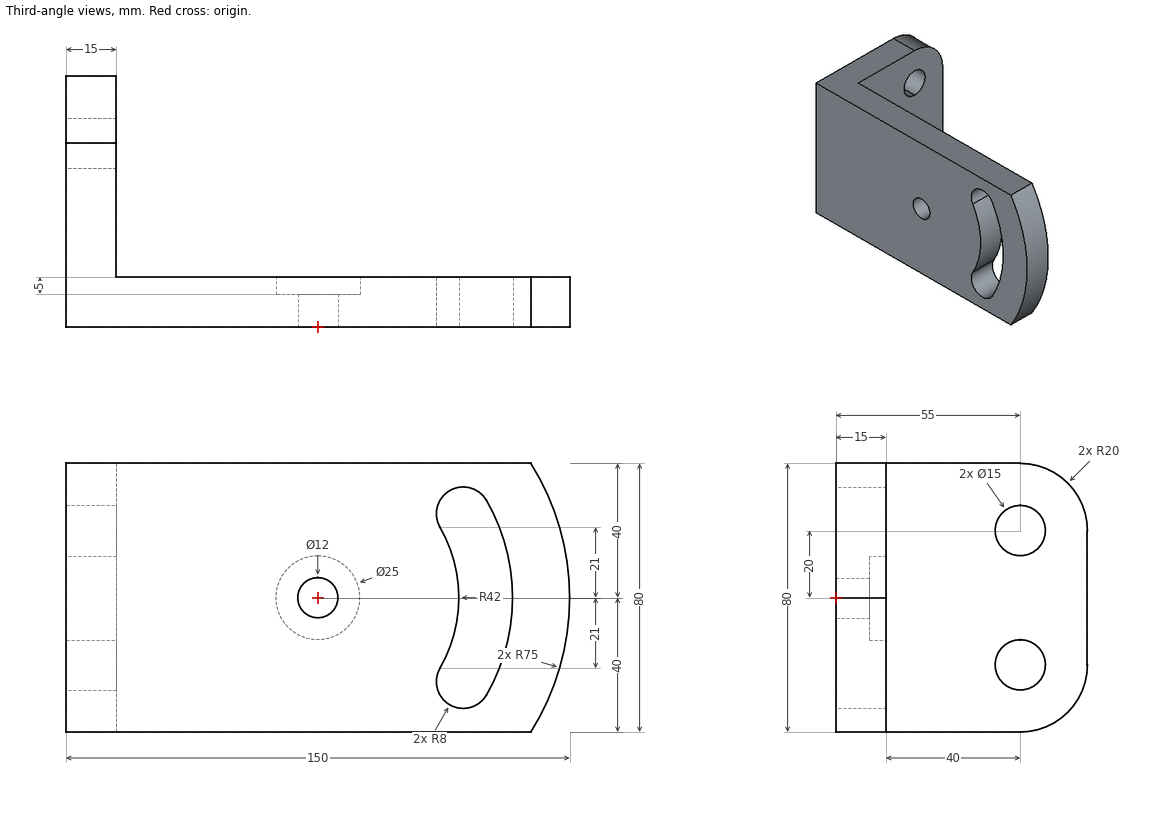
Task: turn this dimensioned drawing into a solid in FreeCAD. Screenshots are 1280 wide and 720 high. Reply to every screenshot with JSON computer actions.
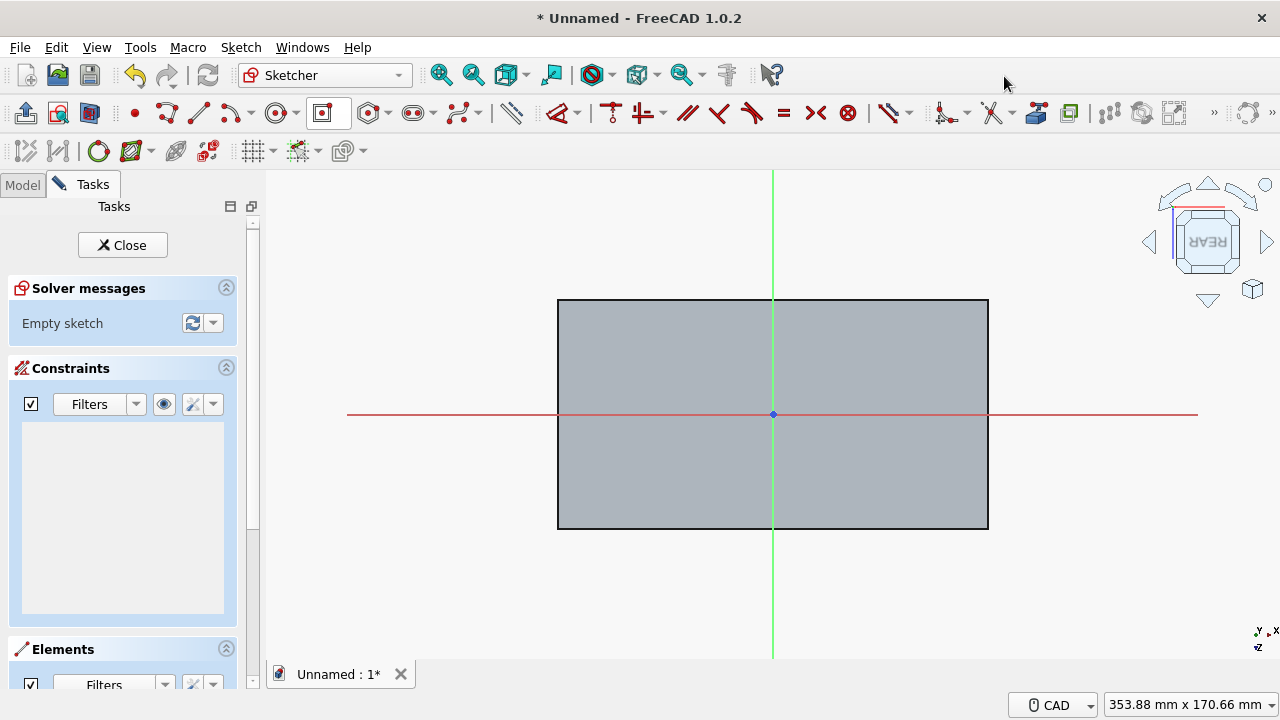
{"action": "left_click", "coordinate": [168, 114]}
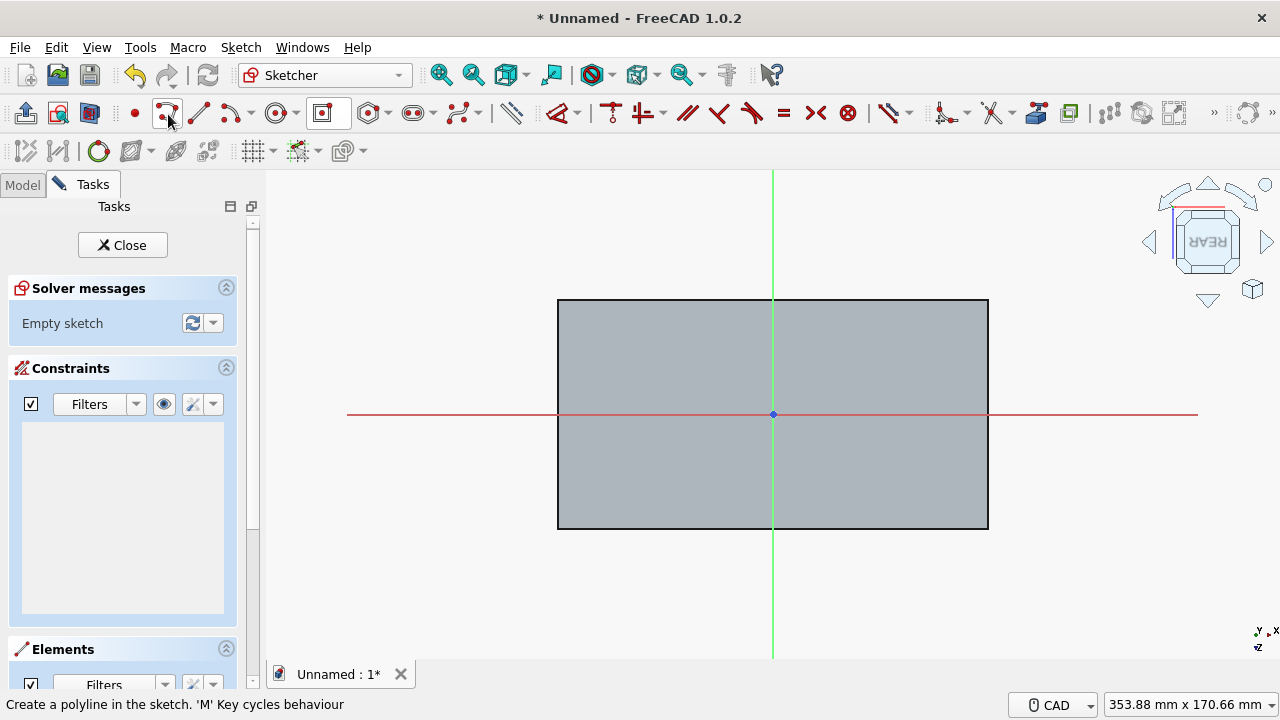
{"action": "left_click", "coordinate": [988, 414]}
{"action": "left_click", "coordinate": [988, 300]}
{"action": "left_click", "coordinate": [955, 300]}
{"action": "right_click", "coordinate": [955, 300]}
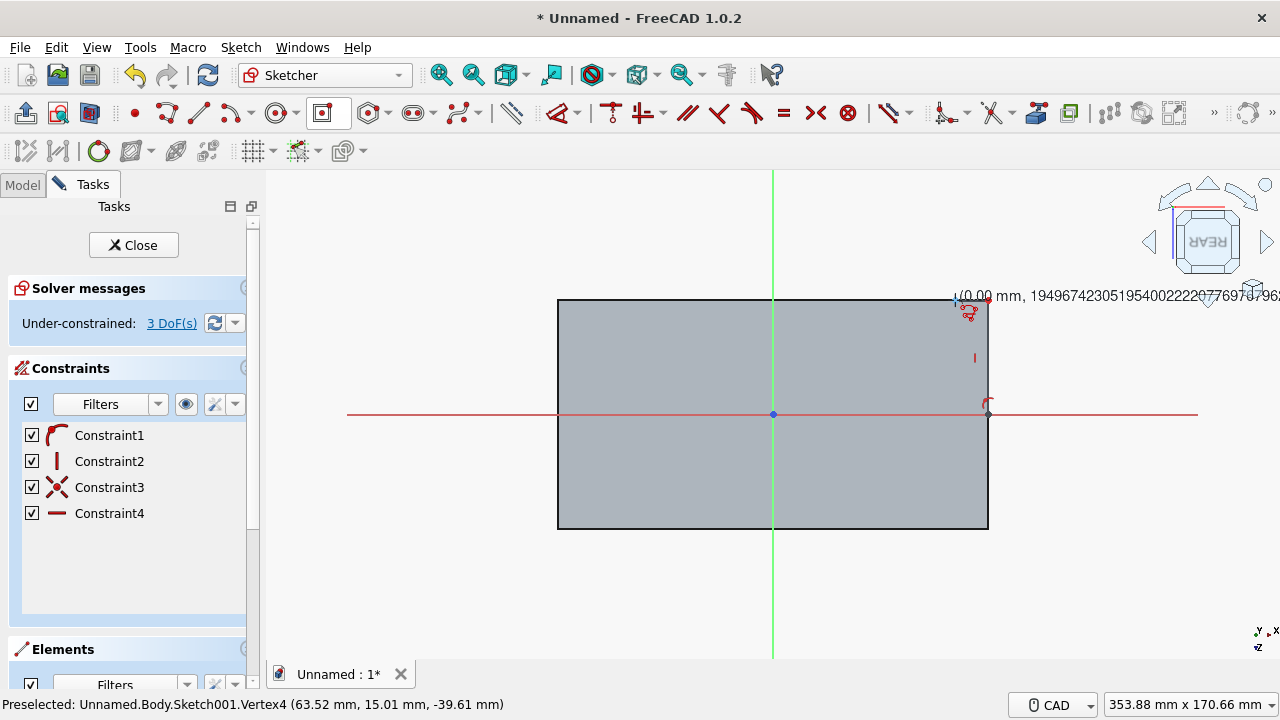
{"action": "key", "text": "g 3 a"}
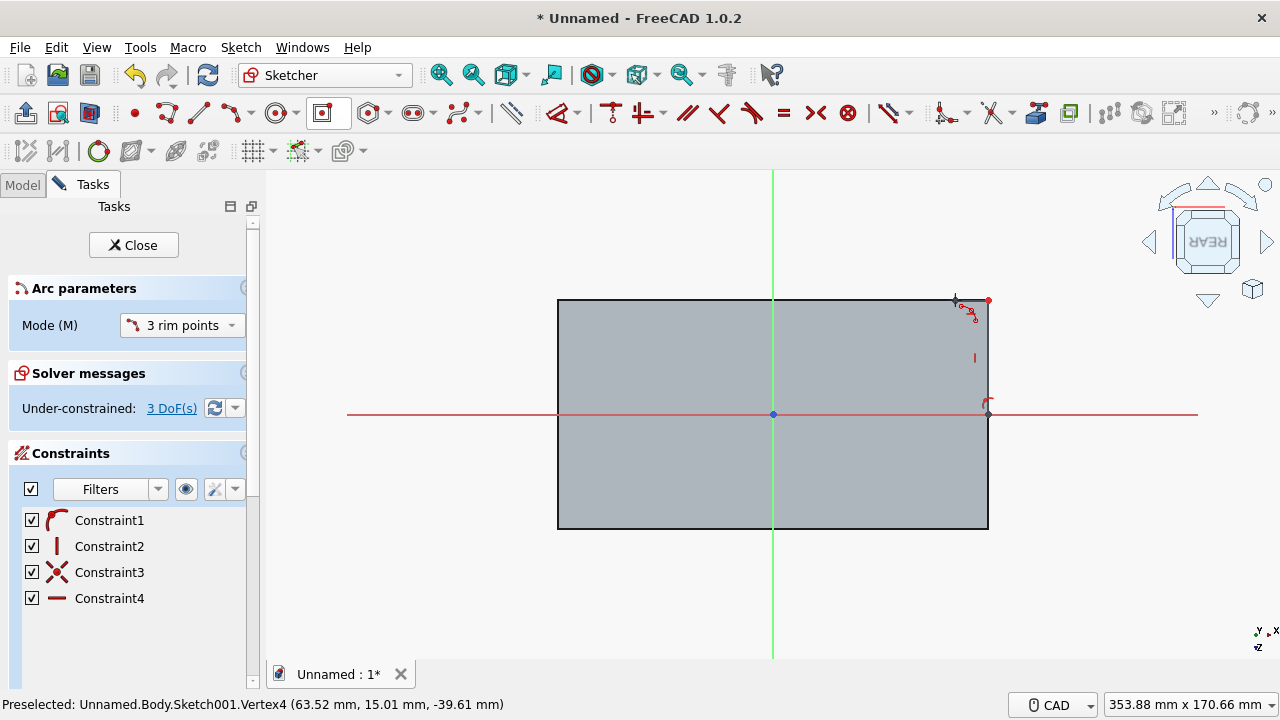
{"action": "left_click", "coordinate": [955, 301]}
{"action": "left_click", "coordinate": [988, 414]}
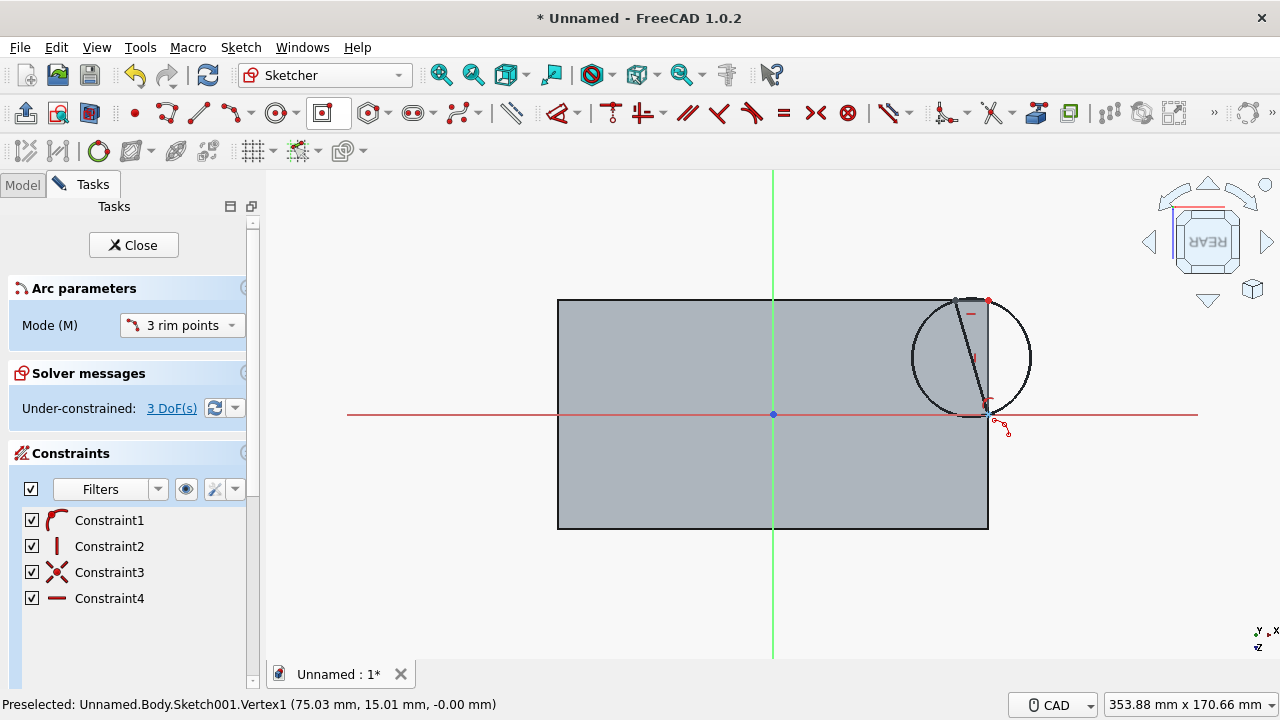
{"action": "scroll", "coordinate": [979, 355], "scroll_direction": "up", "scroll_amount": 4}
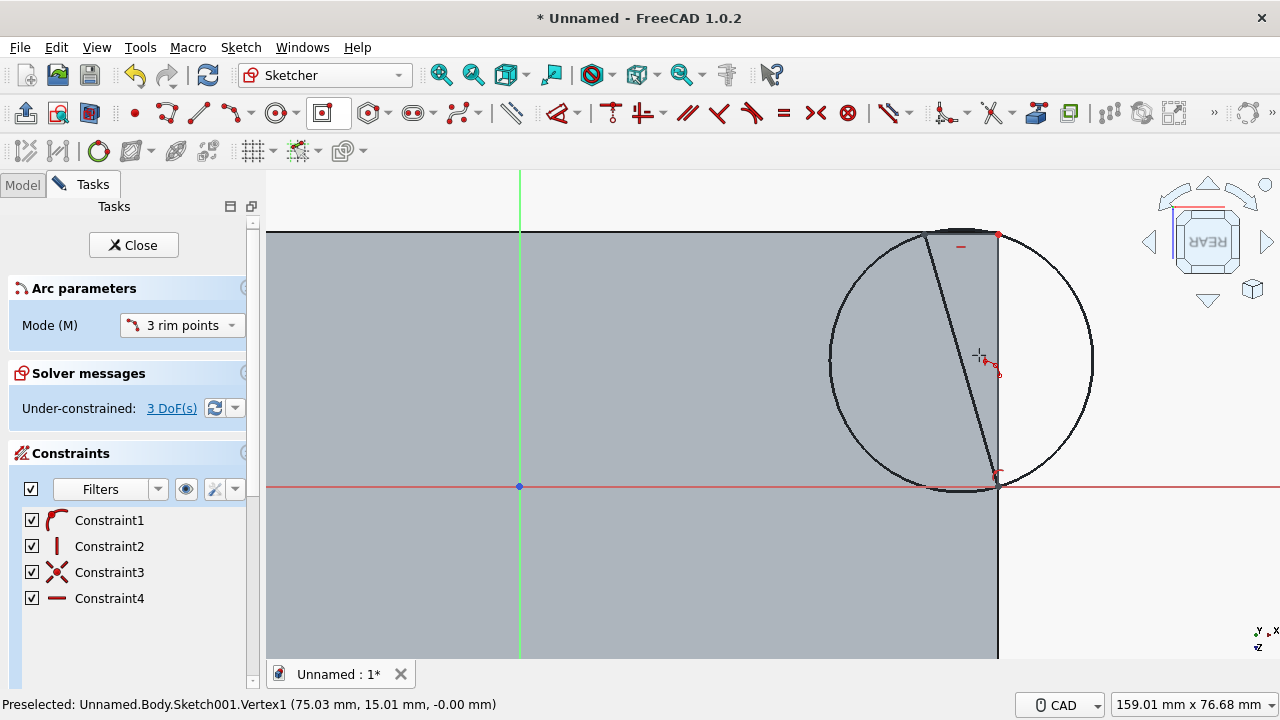
{"action": "left_click", "coordinate": [979, 354]}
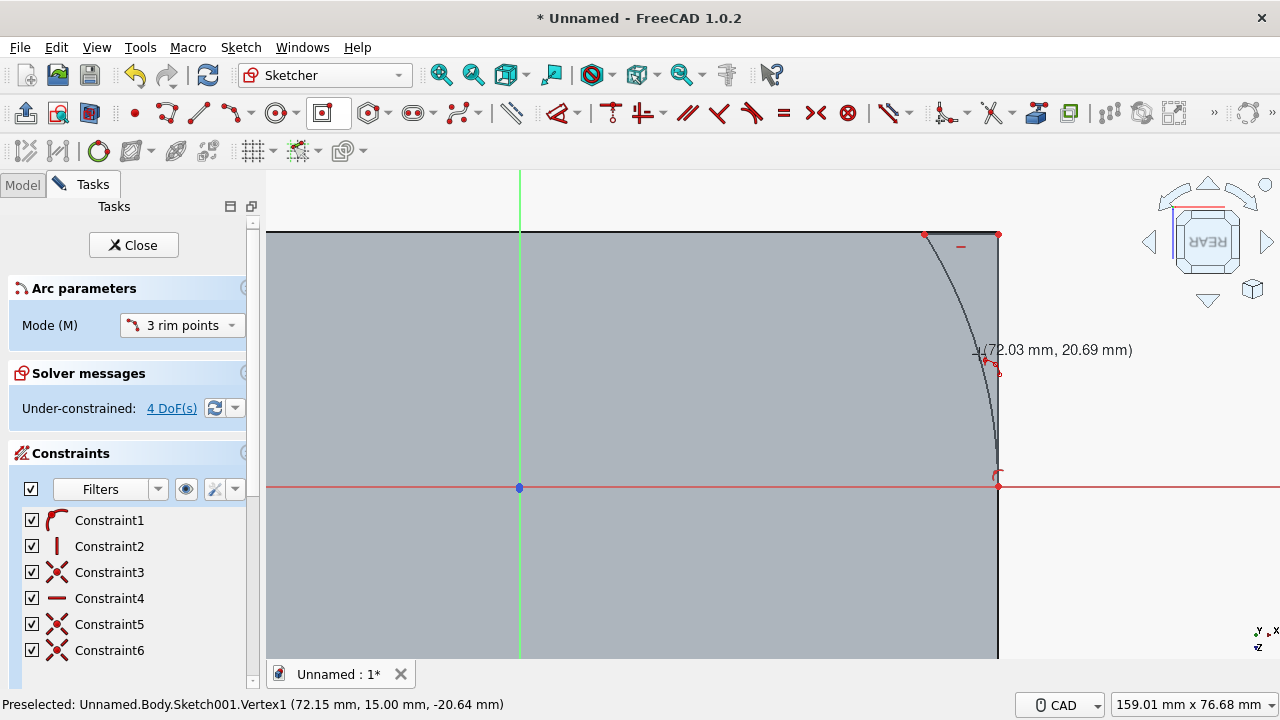
{"action": "left_click", "coordinate": [168, 114]}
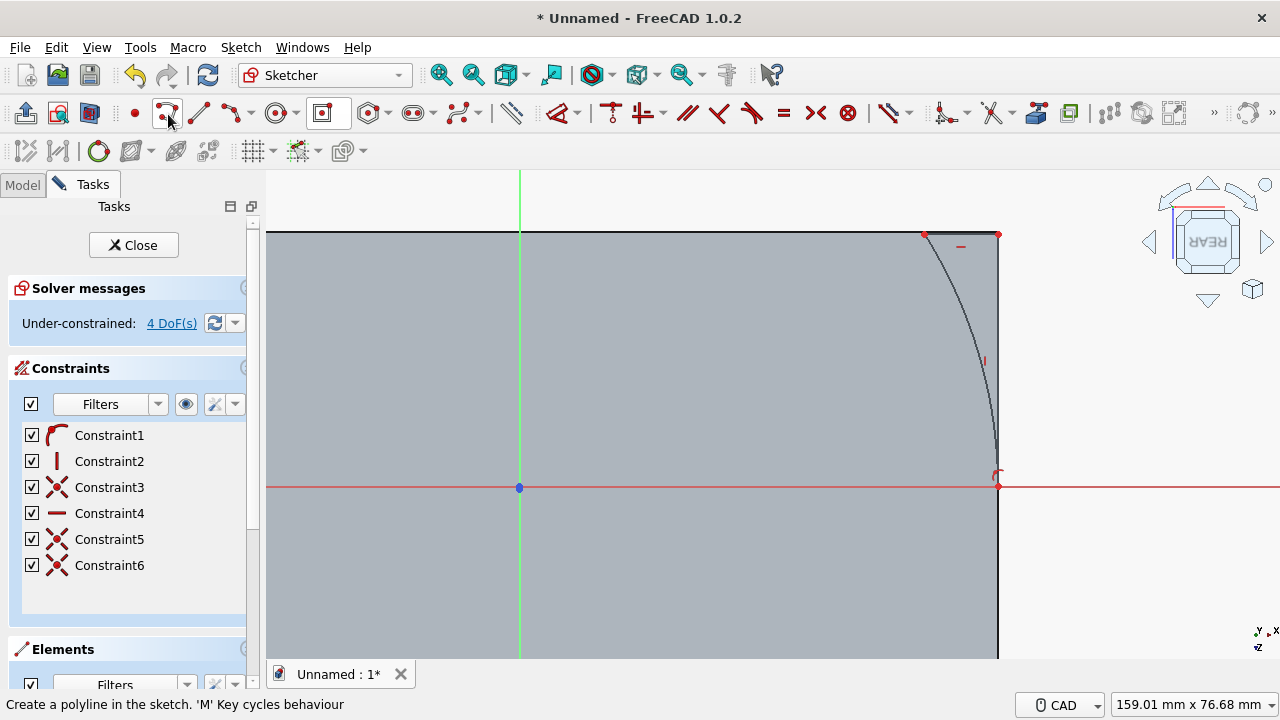
{"action": "scroll", "coordinate": [638, 326], "scroll_direction": "down", "scroll_amount": 3}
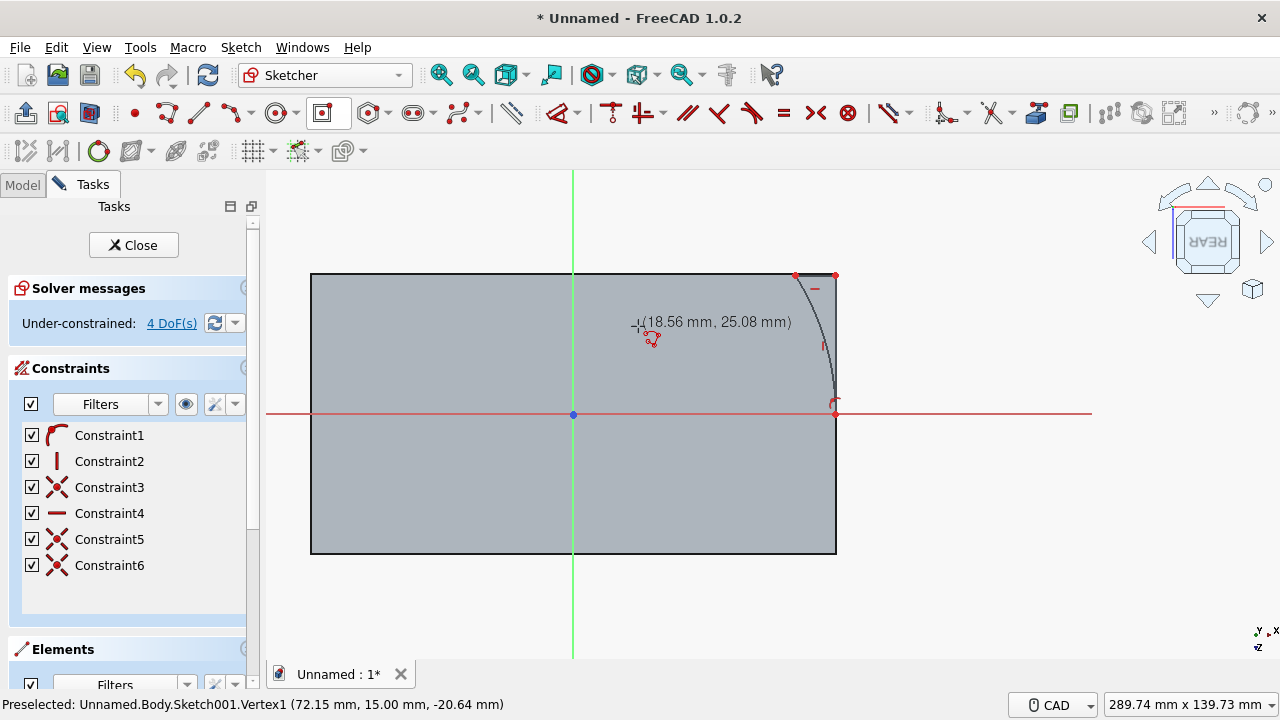
{"action": "left_click", "coordinate": [795, 554]}
{"action": "left_click", "coordinate": [836, 554]}
{"action": "left_click", "coordinate": [836, 414]}
{"action": "right_click", "coordinate": [836, 554]}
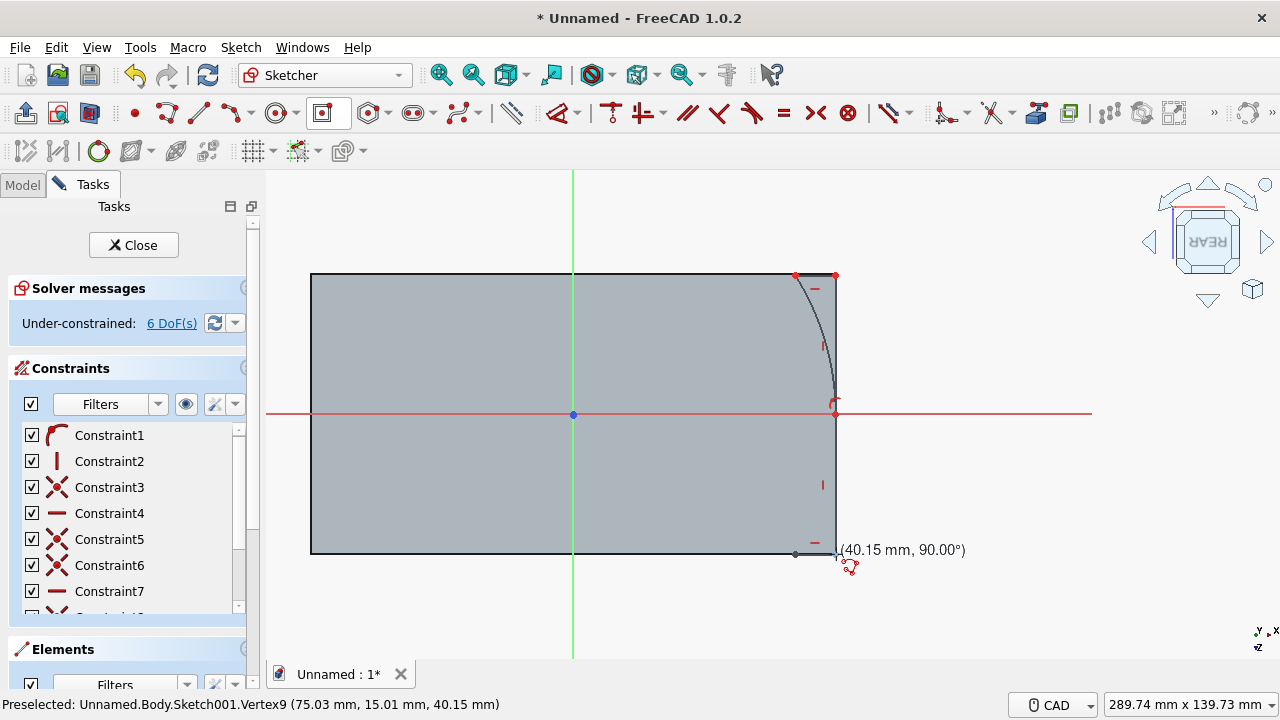
{"action": "left_click", "coordinate": [232, 114]}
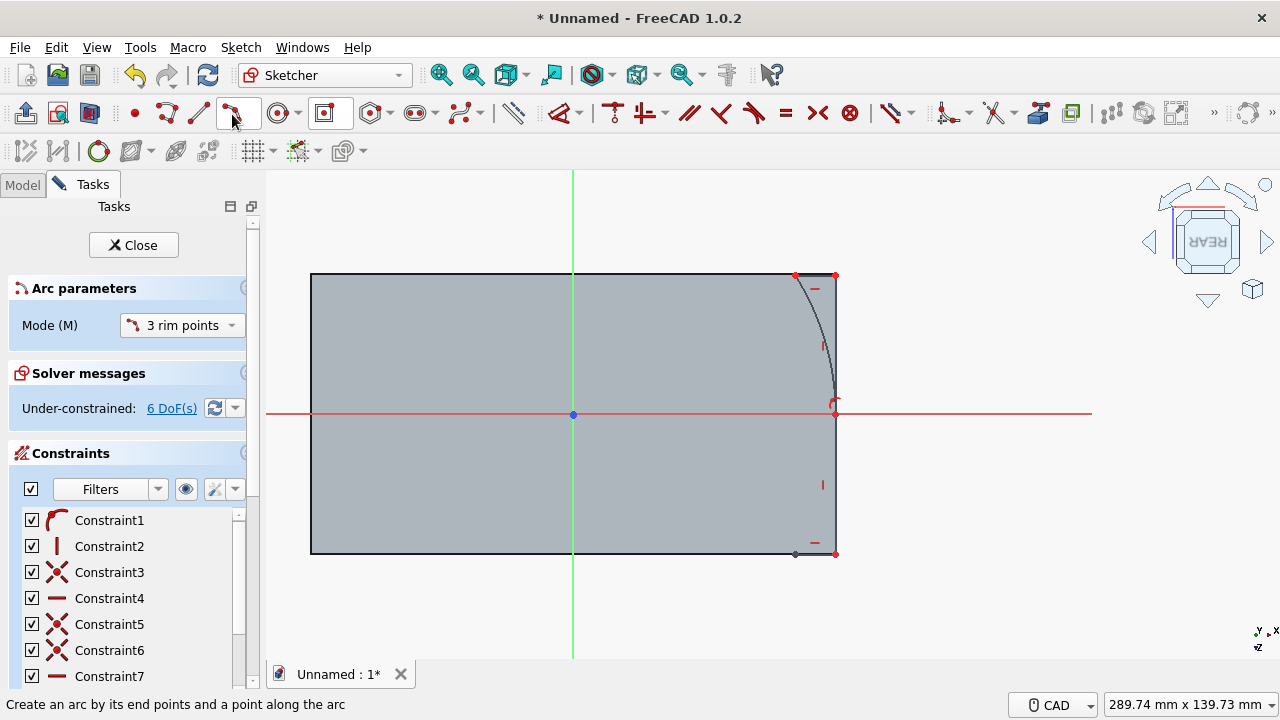
{"action": "left_click", "coordinate": [836, 414]}
{"action": "left_click", "coordinate": [795, 555]}